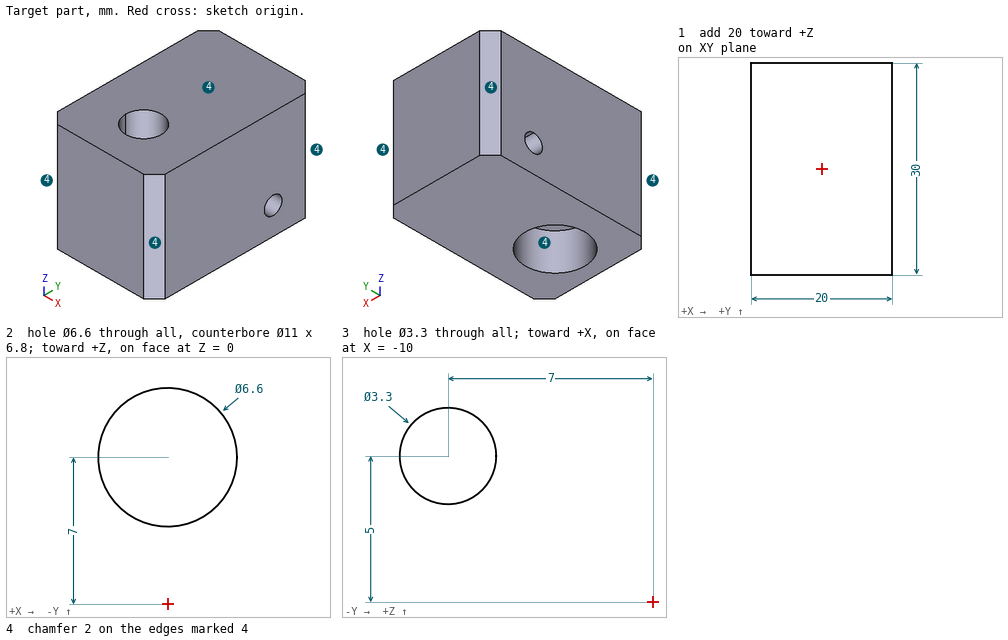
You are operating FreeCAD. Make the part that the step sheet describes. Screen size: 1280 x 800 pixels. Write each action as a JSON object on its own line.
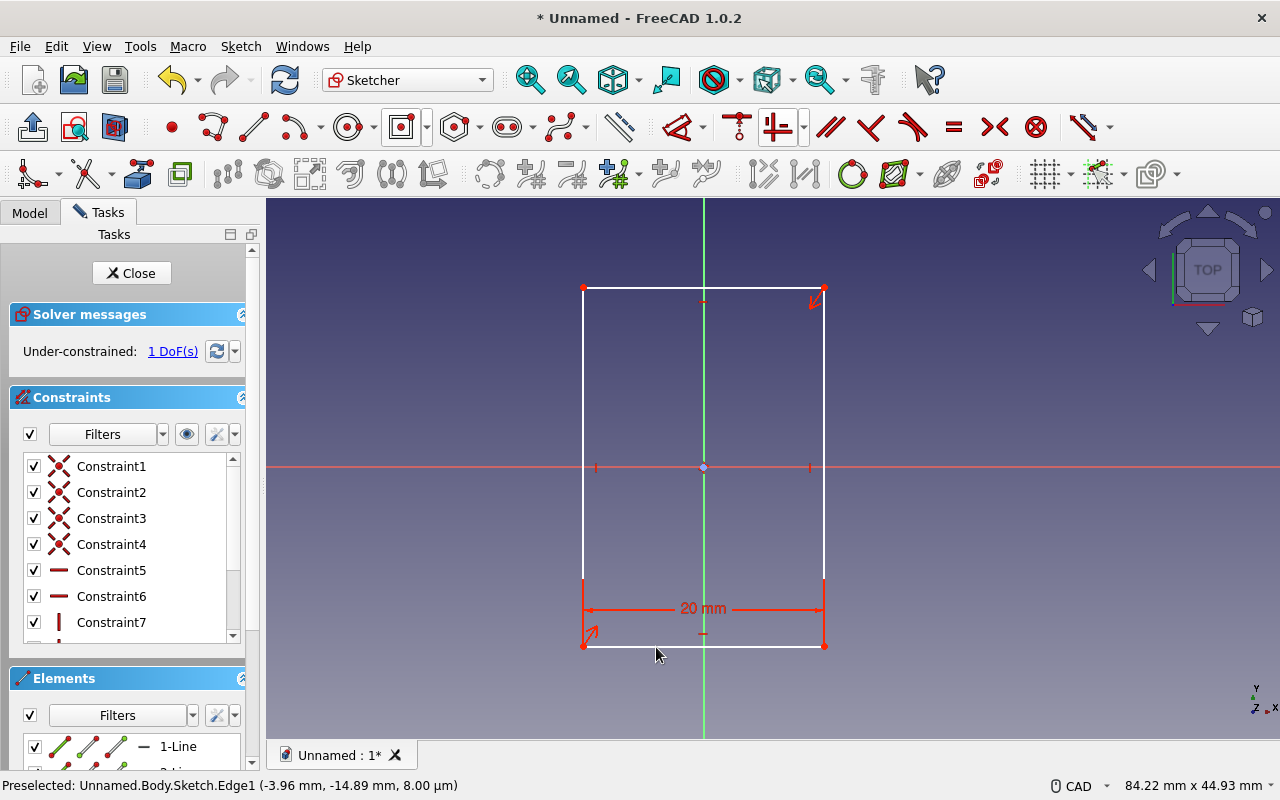
{"action": "left_click", "coordinate": [824, 539]}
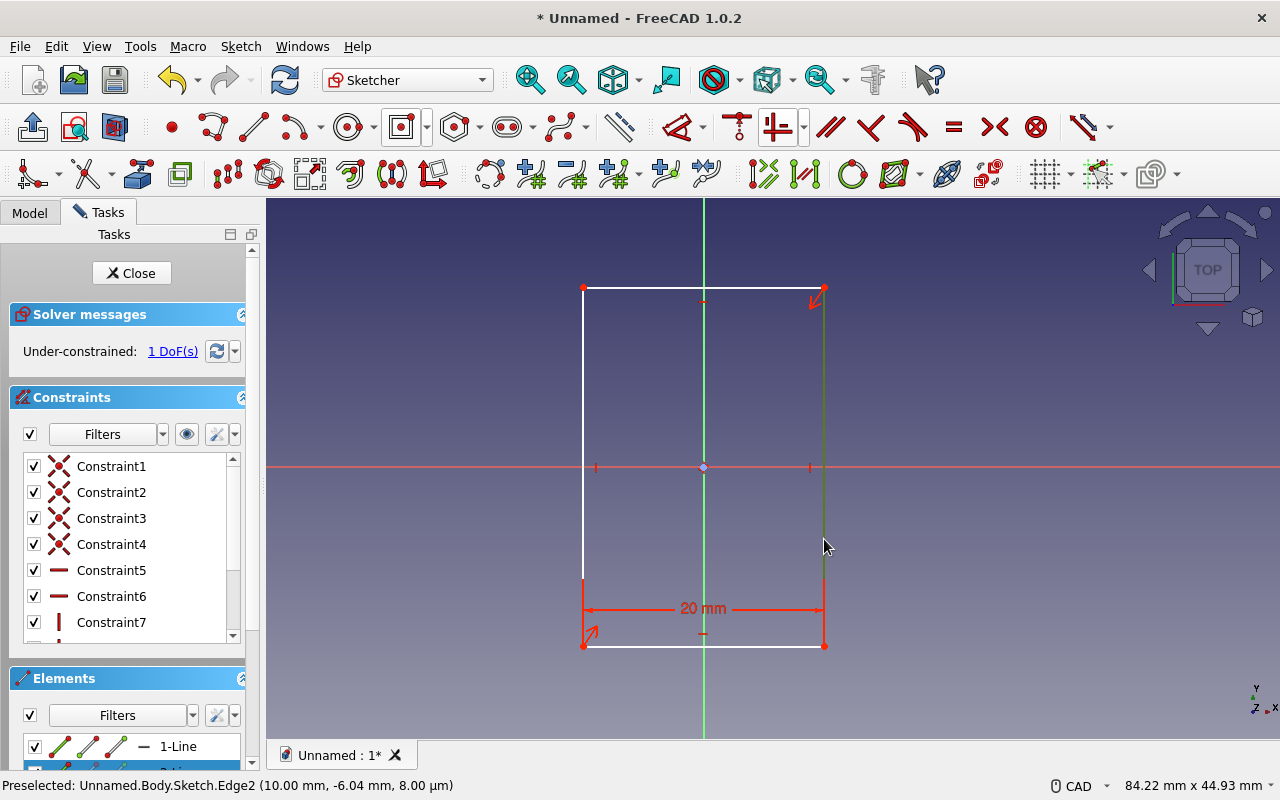
{"action": "key", "text": "i"}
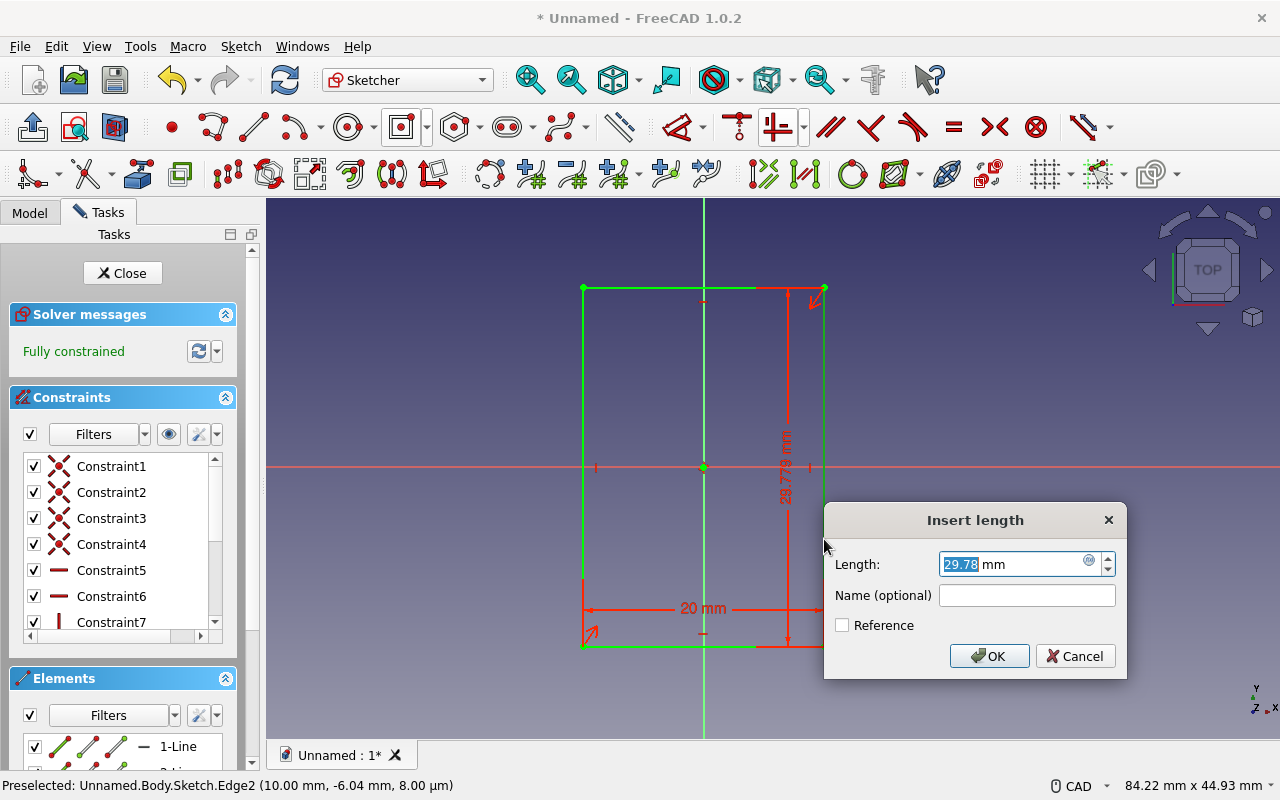
{"action": "type", "text": "30"}
{"action": "key", "text": "Return"}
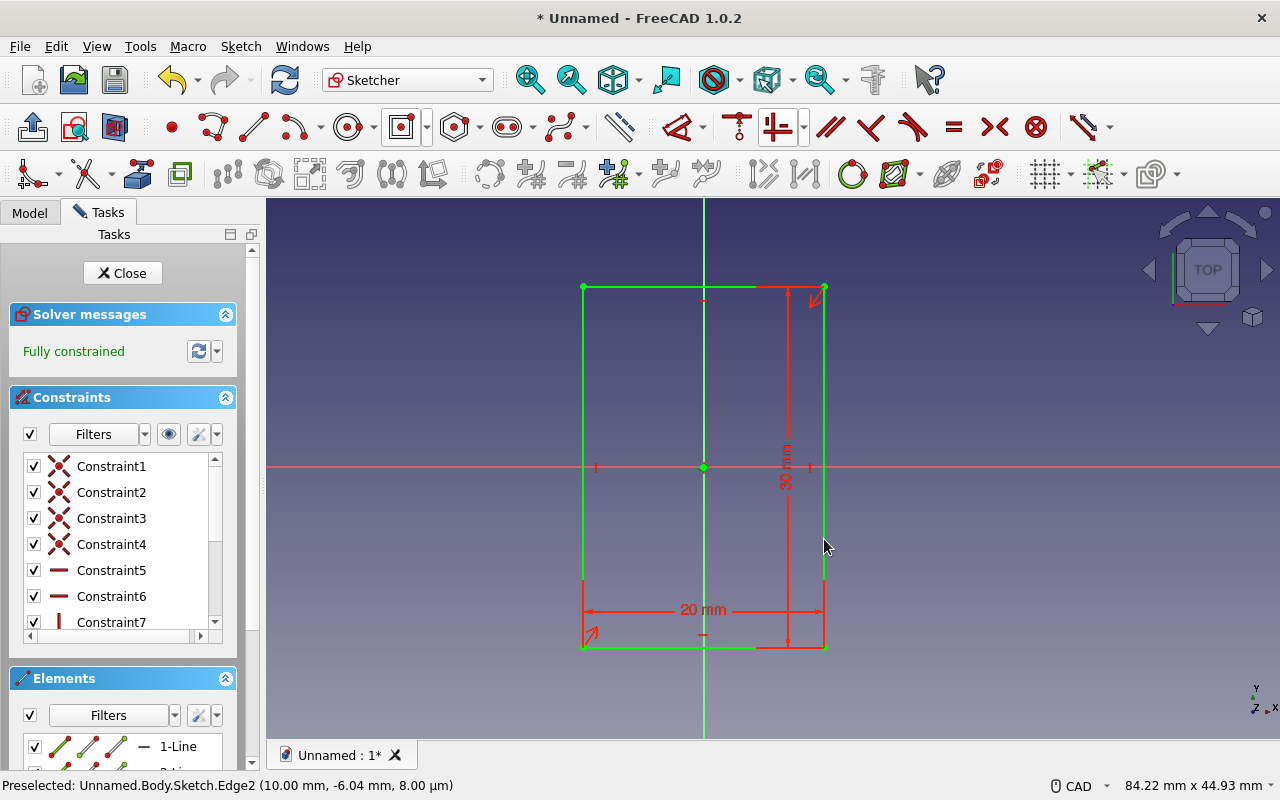
{"action": "left_click", "coordinate": [123, 273]}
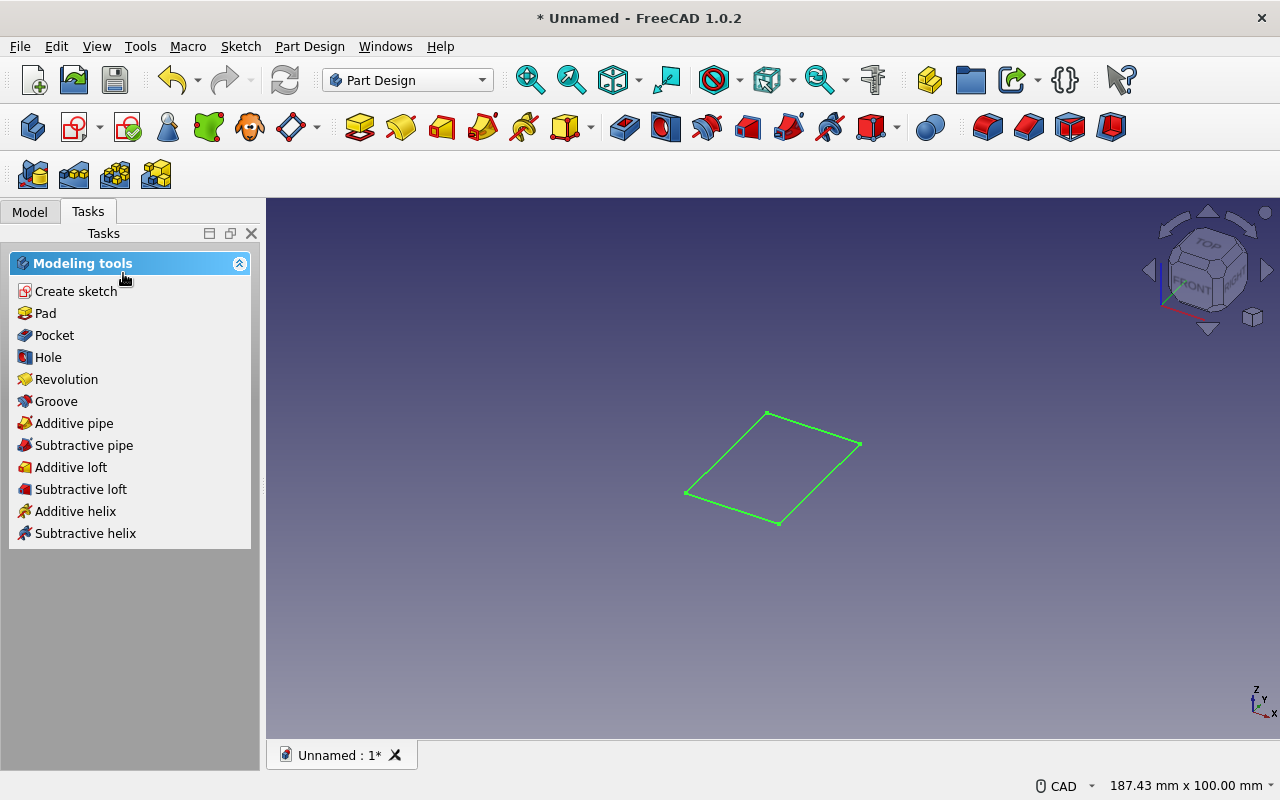
{"action": "left_click", "coordinate": [360, 128]}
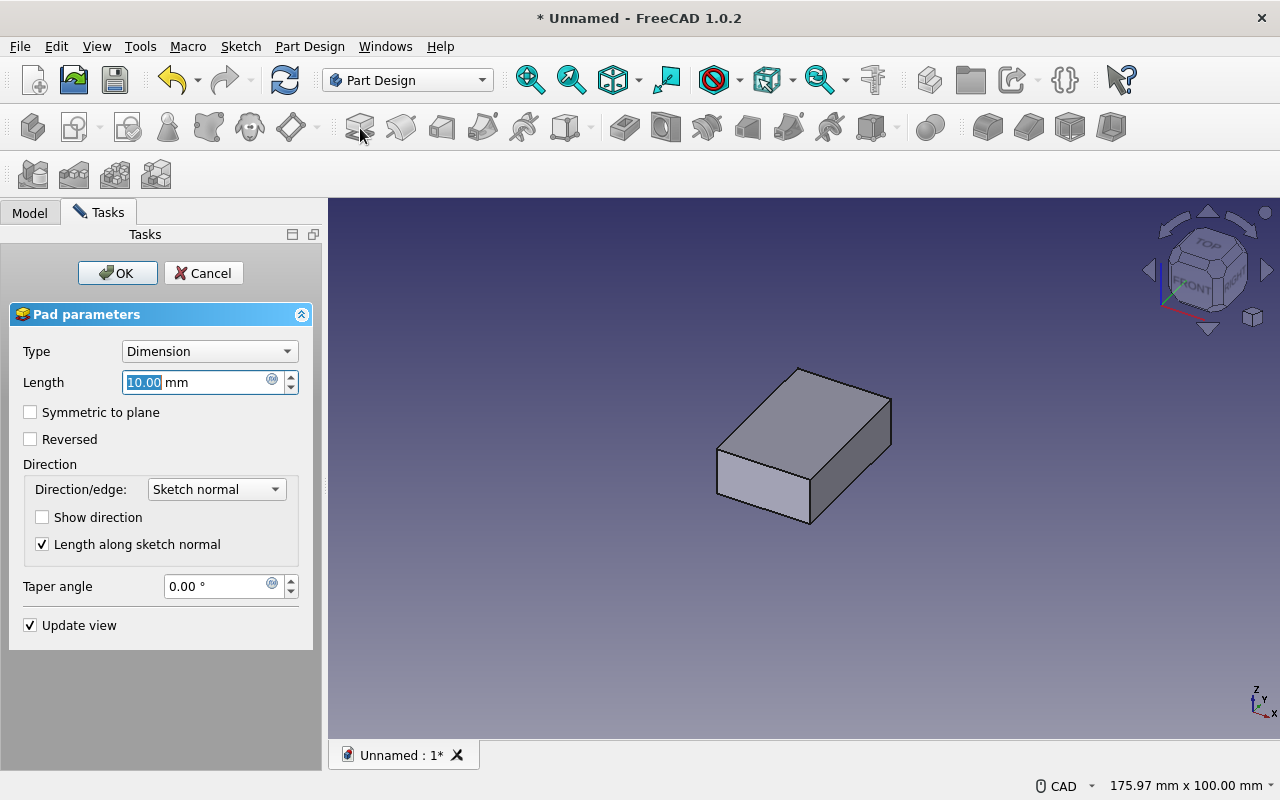
{"action": "type", "text": "20"}
{"action": "key", "text": "Tab"}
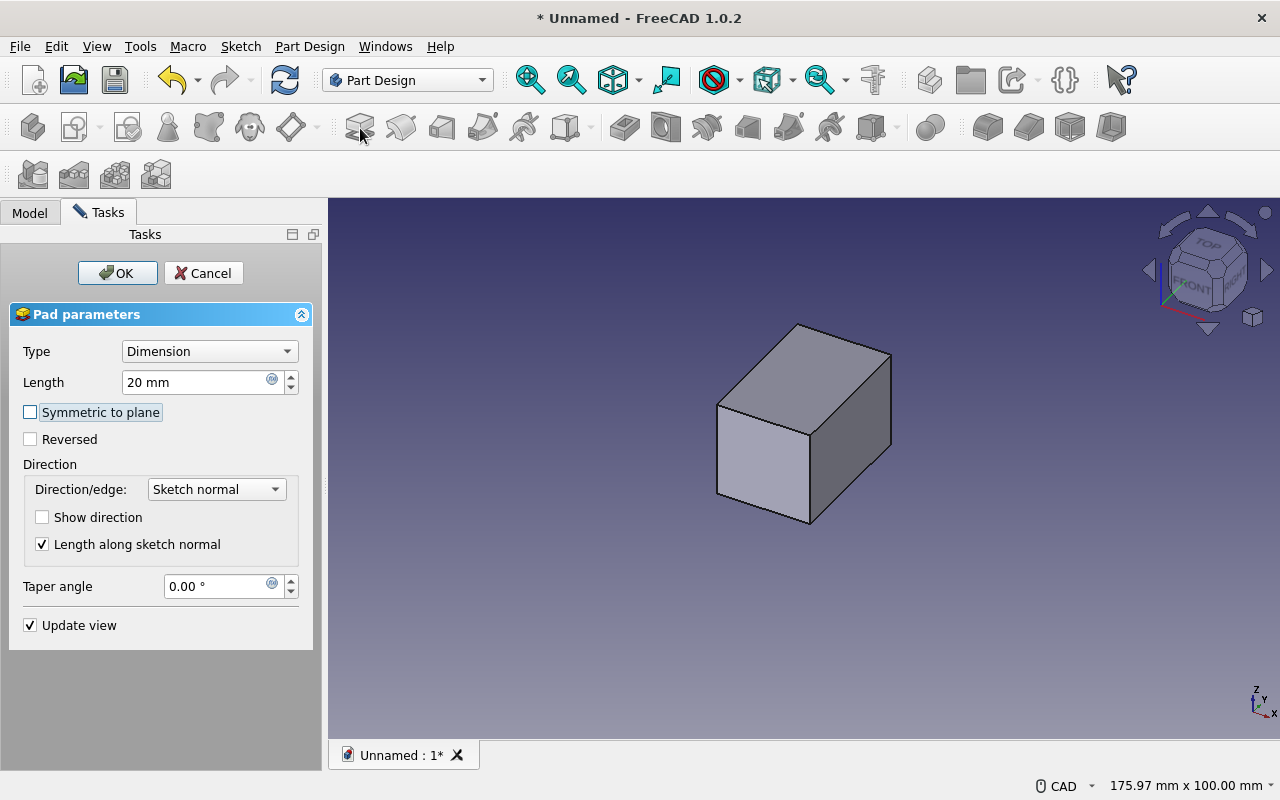
{"action": "left_click", "coordinate": [118, 273]}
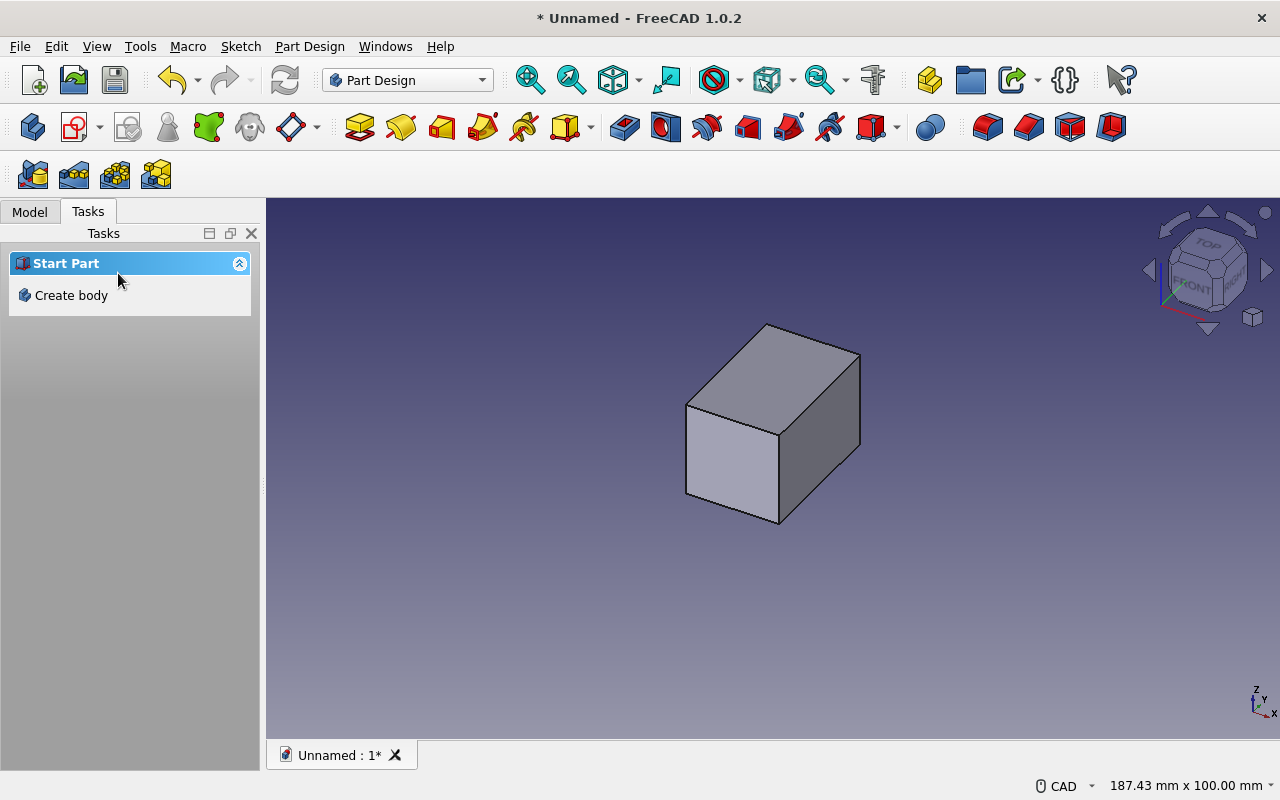
{"action": "key", "text": "v f"}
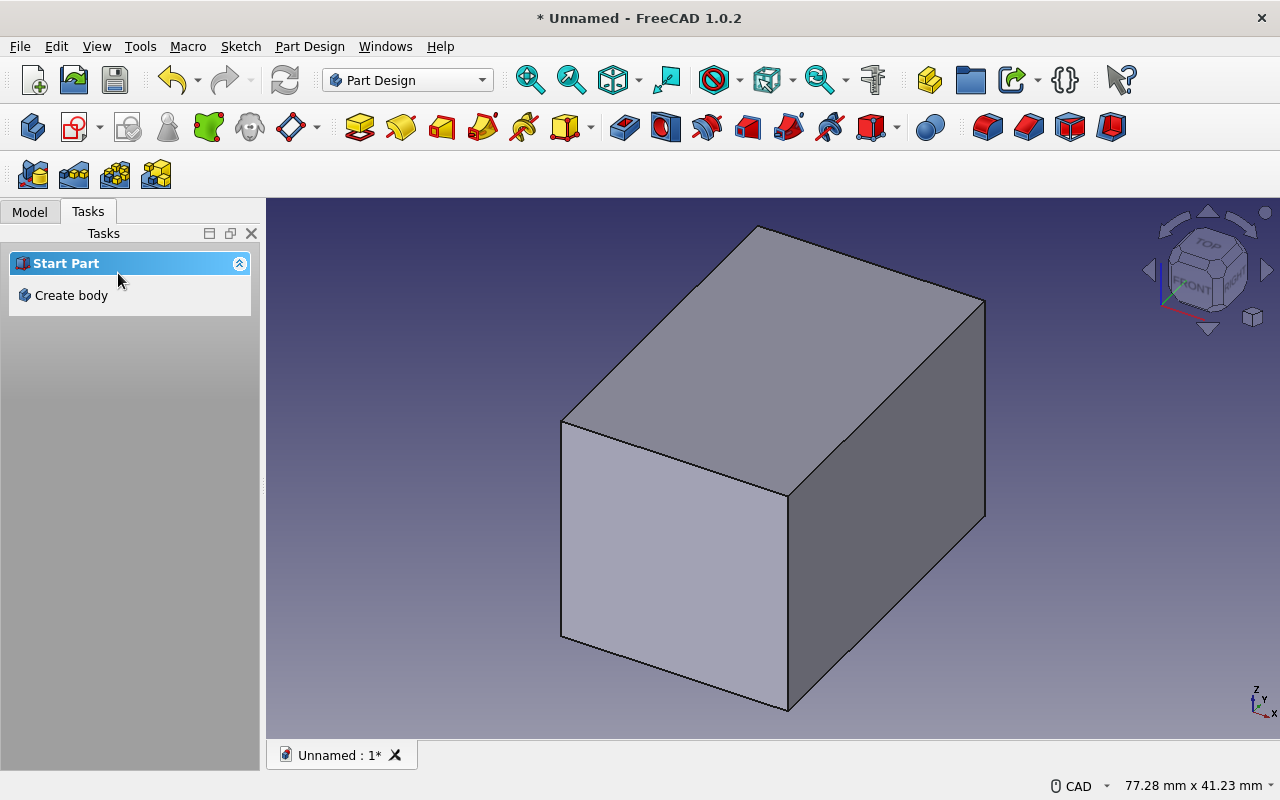
{"action": "key", "text": "5"}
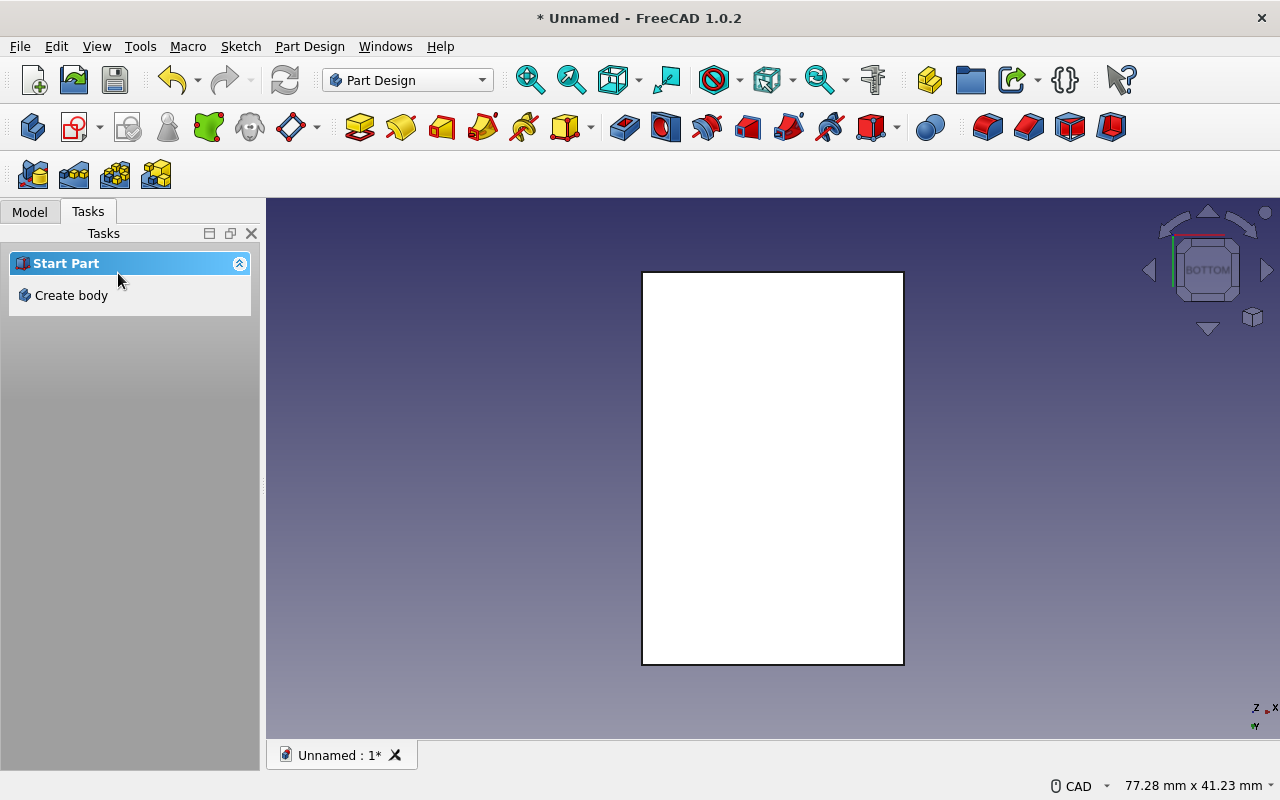
{"action": "left_click", "coordinate": [773, 524]}